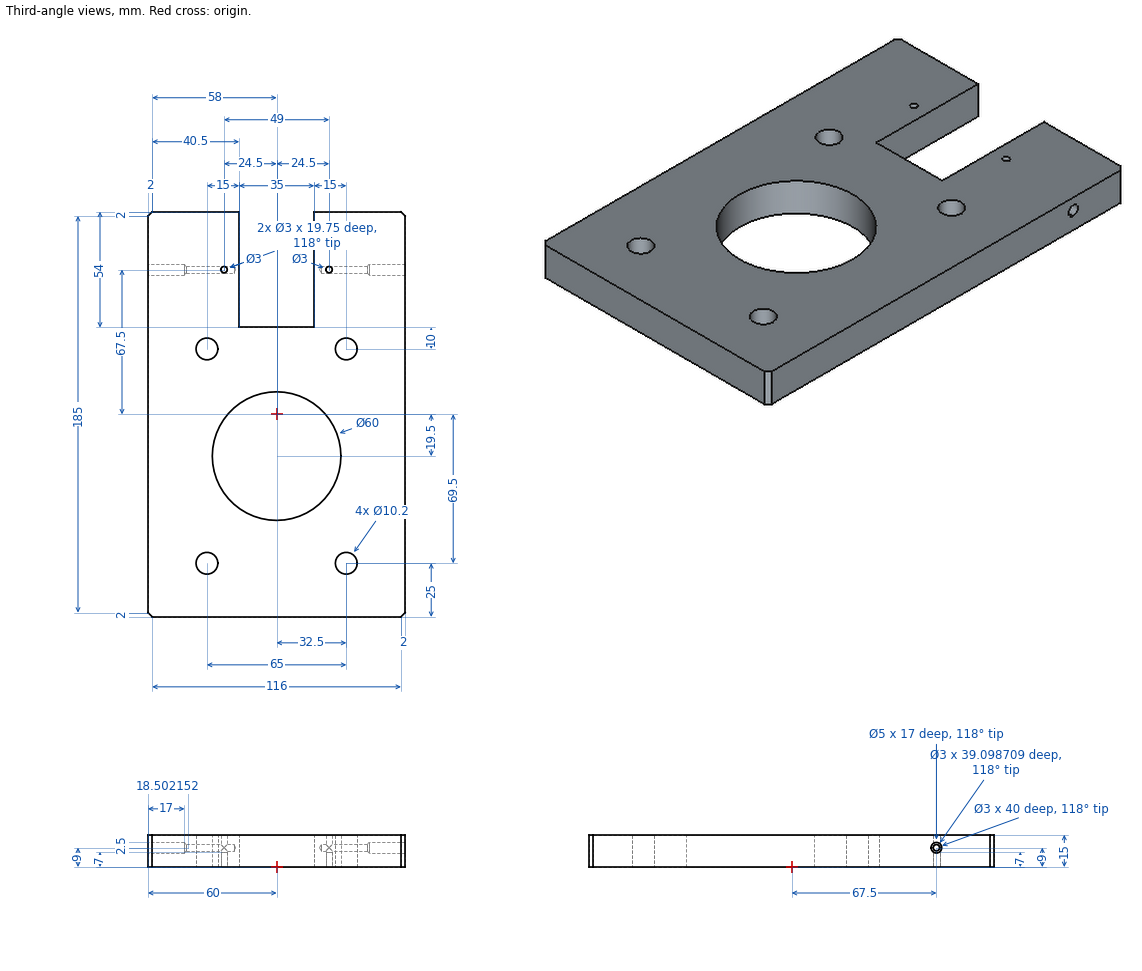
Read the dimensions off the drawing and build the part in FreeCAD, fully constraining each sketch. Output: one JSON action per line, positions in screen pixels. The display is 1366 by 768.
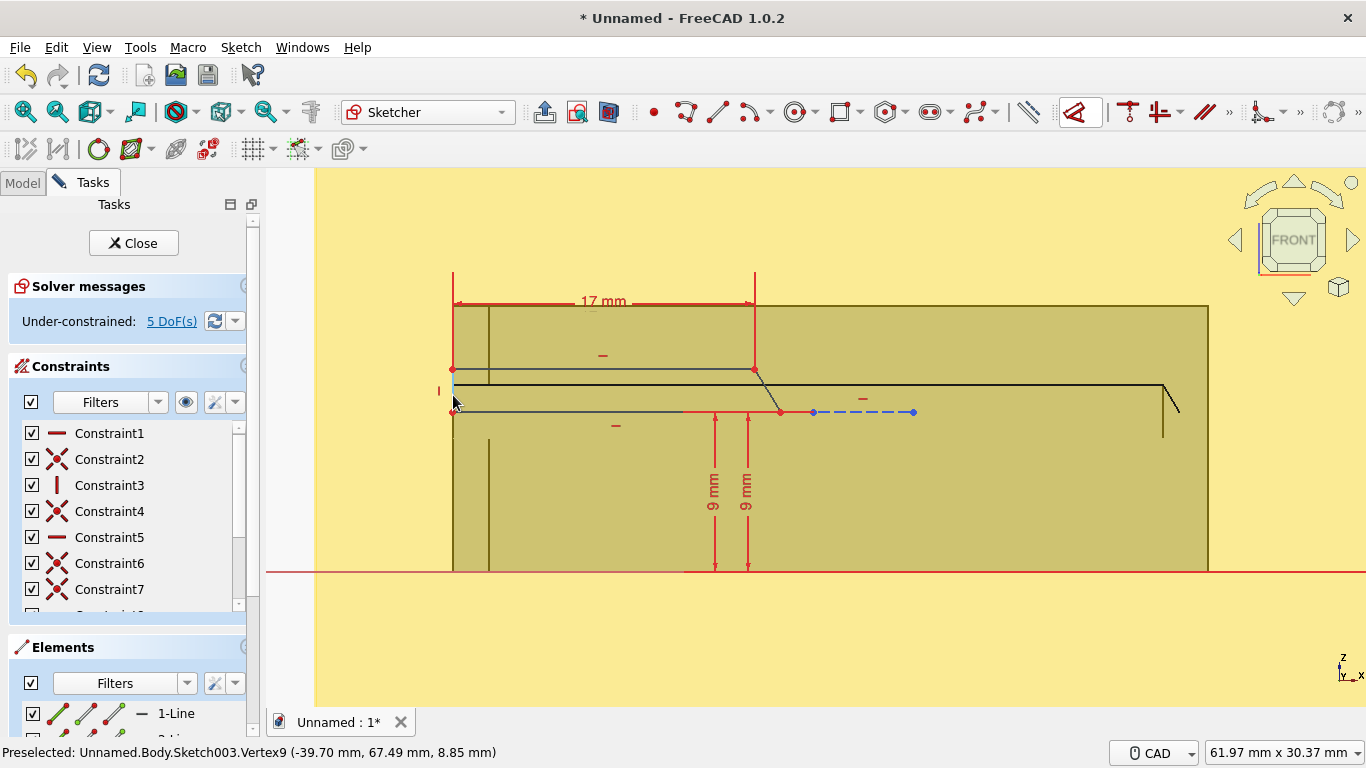
{"action": "left_click", "coordinate": [453, 395]}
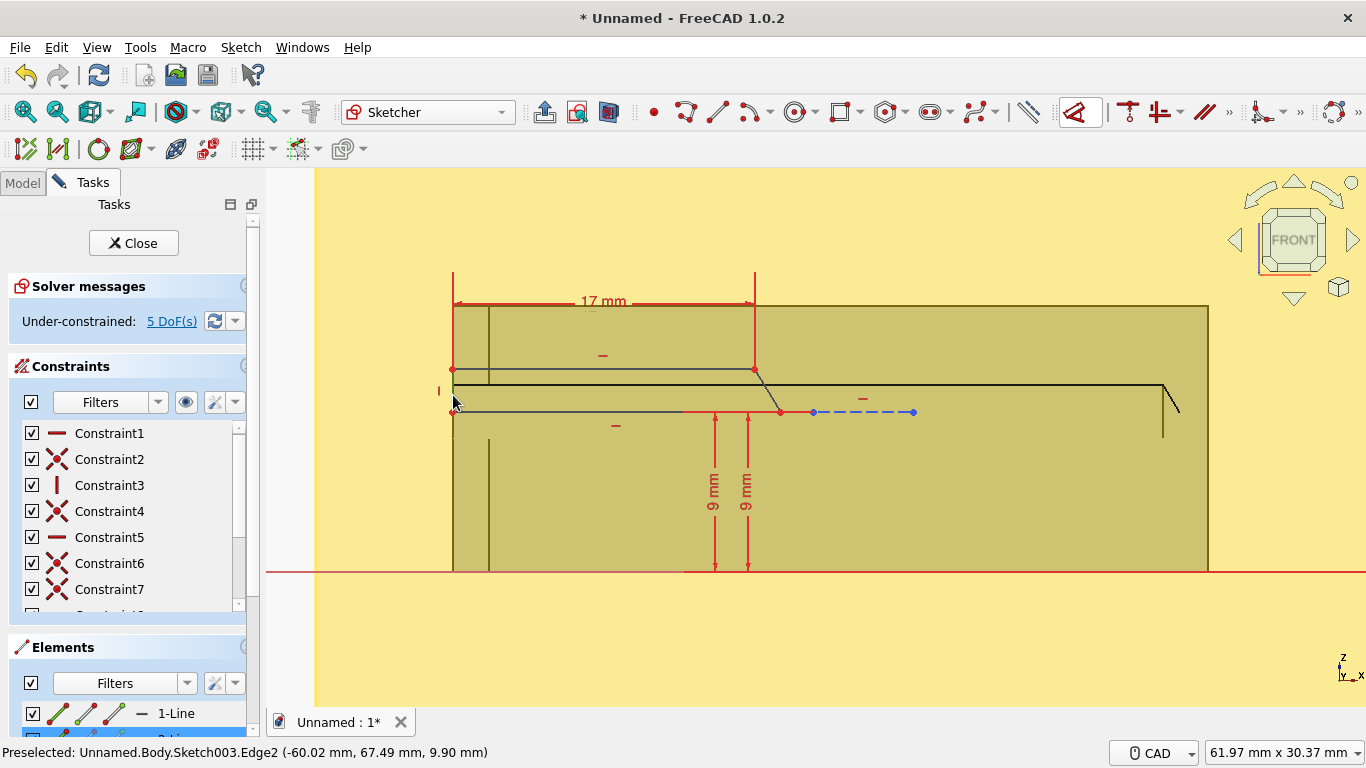
{"action": "left_click", "coordinate": [1096, 112]}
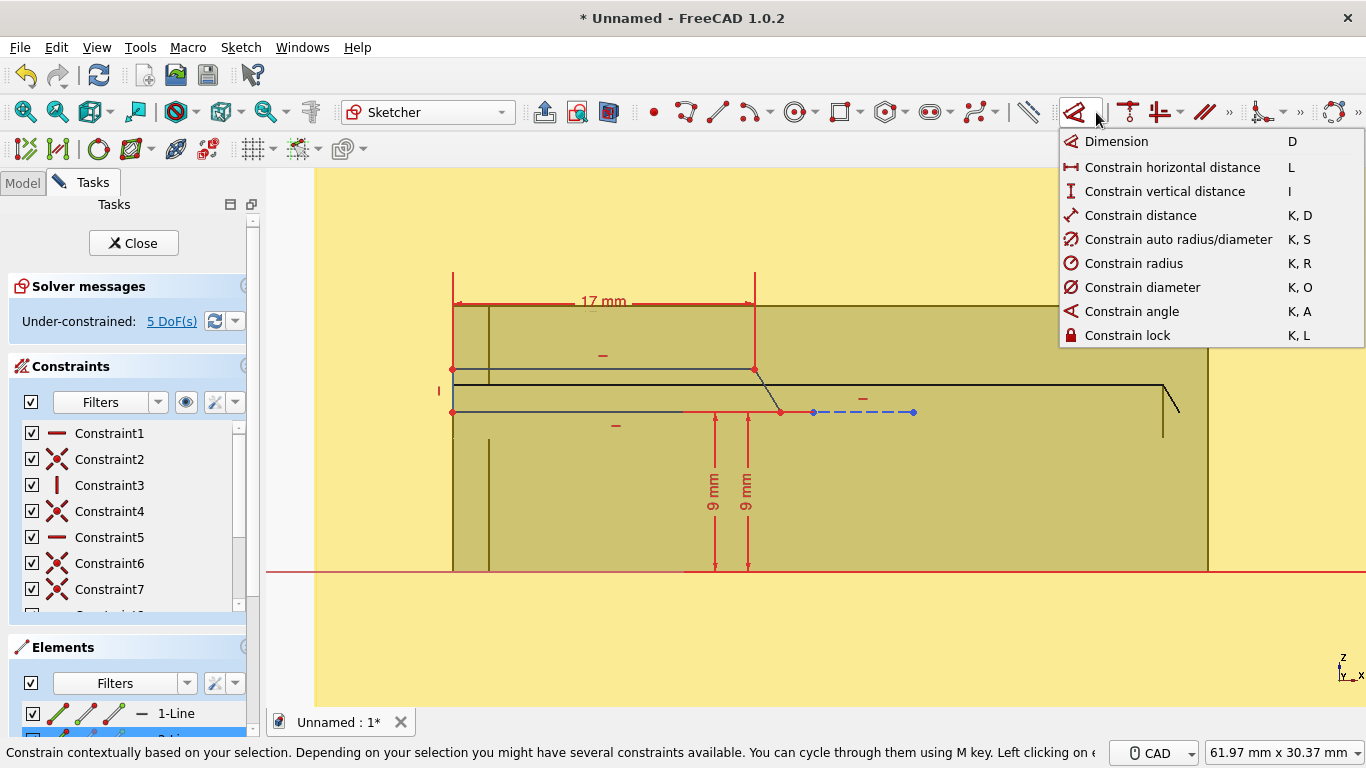
{"action": "left_click", "coordinate": [1212, 191]}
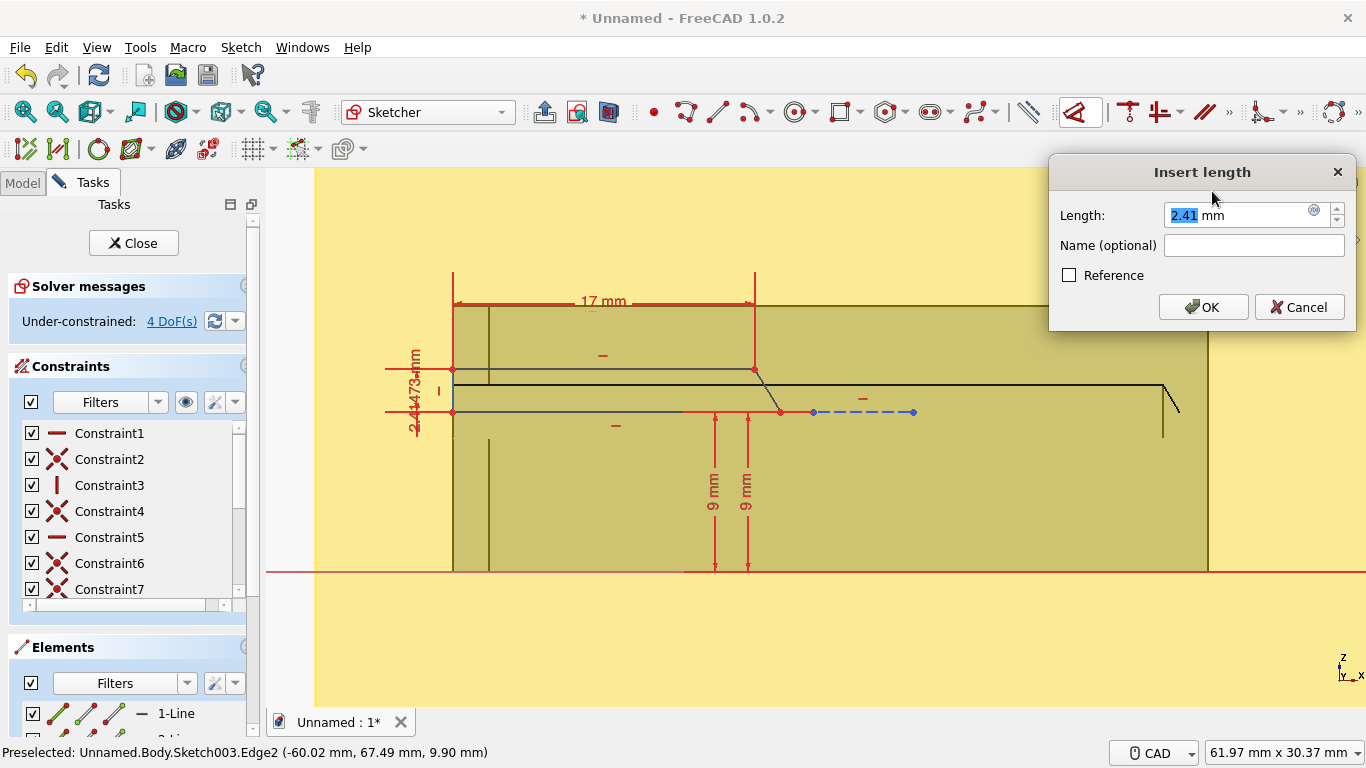
{"action": "type", "text": "2.5"}
{"action": "key", "text": "Return"}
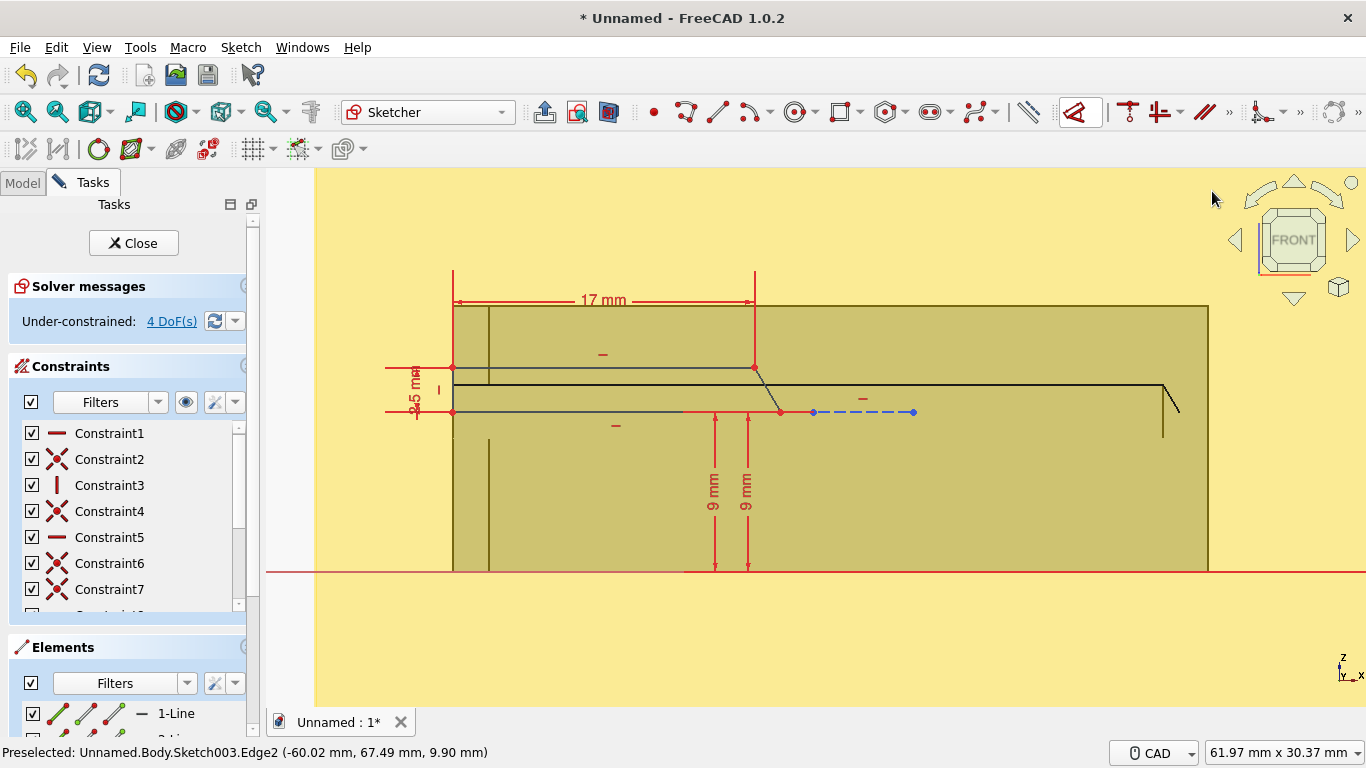
{"action": "left_click", "coordinate": [453, 412]}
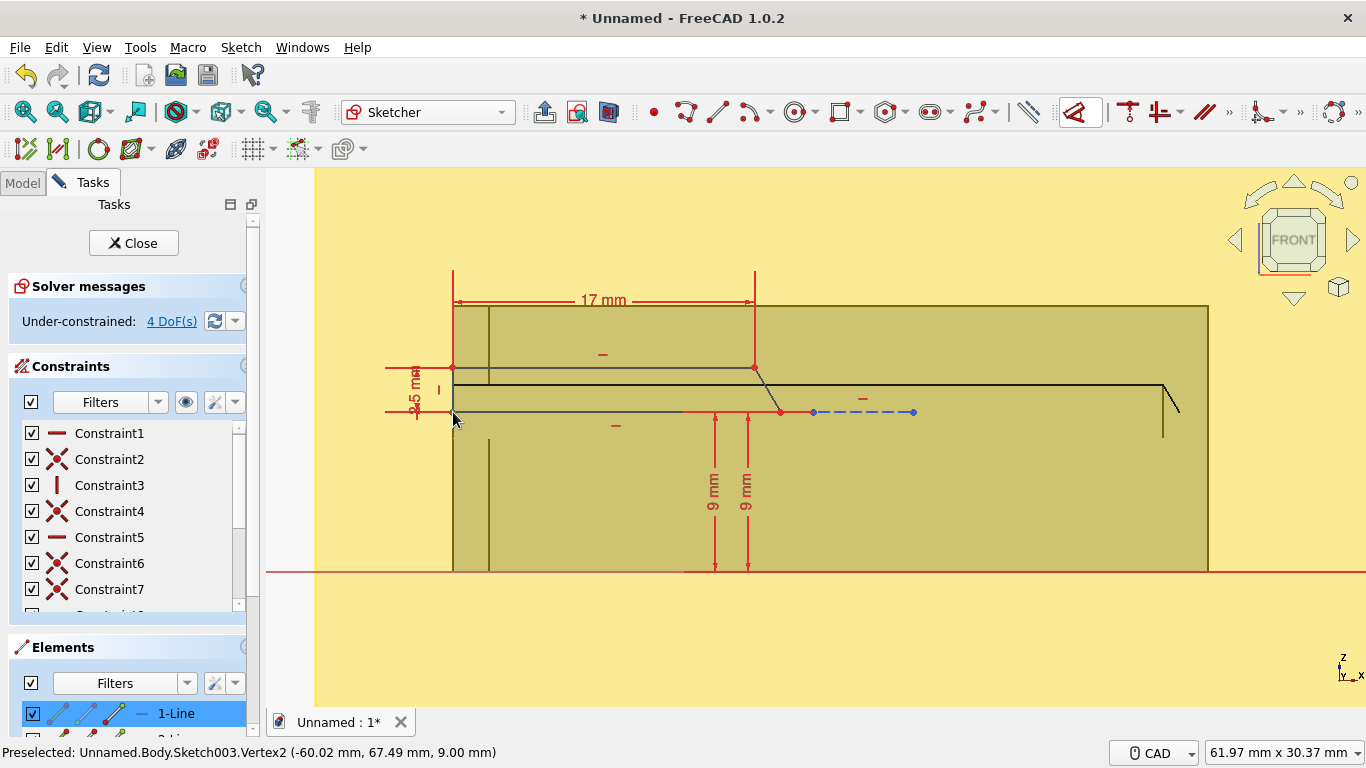
{"action": "left_click", "coordinate": [1096, 112]}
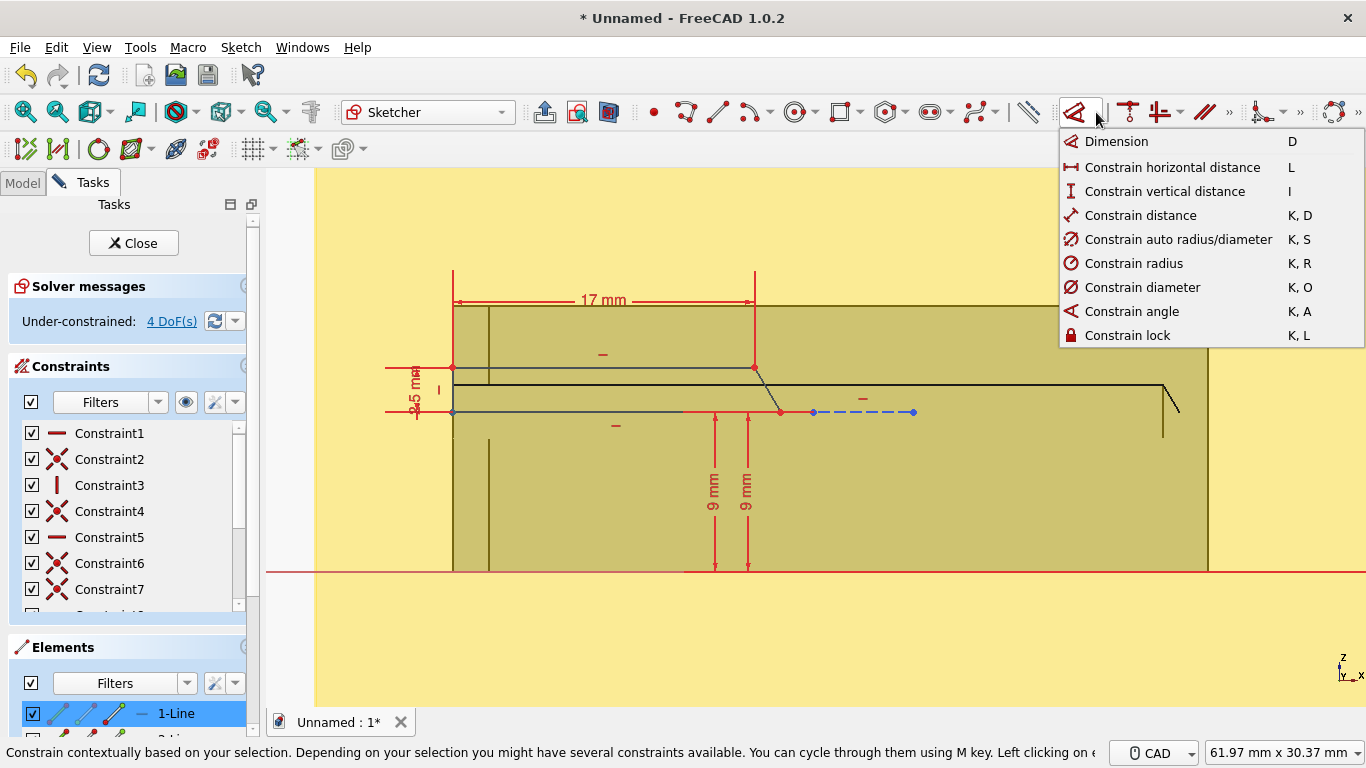
{"action": "left_click", "coordinate": [1212, 167]}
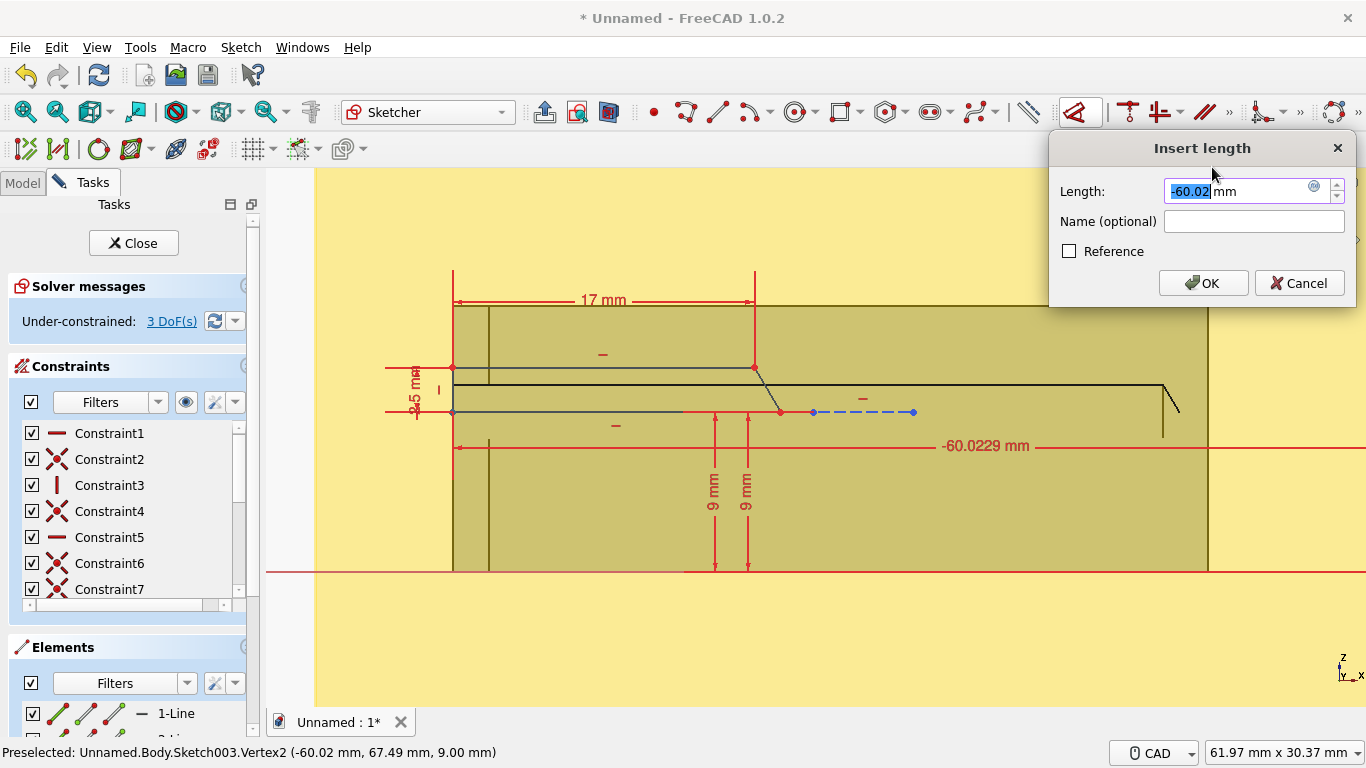
{"action": "type", "text": "-60"}
{"action": "key", "text": "Return"}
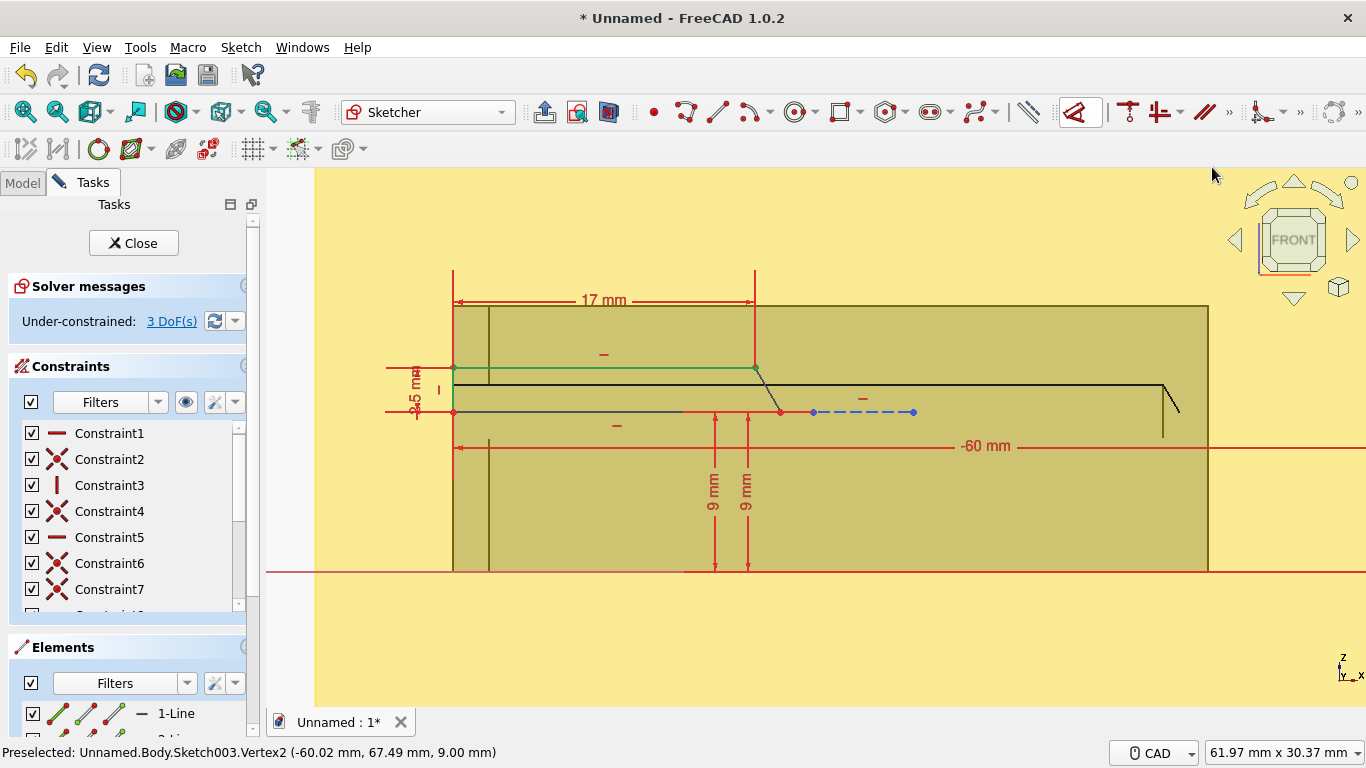
{"action": "left_click", "coordinate": [683, 412]}